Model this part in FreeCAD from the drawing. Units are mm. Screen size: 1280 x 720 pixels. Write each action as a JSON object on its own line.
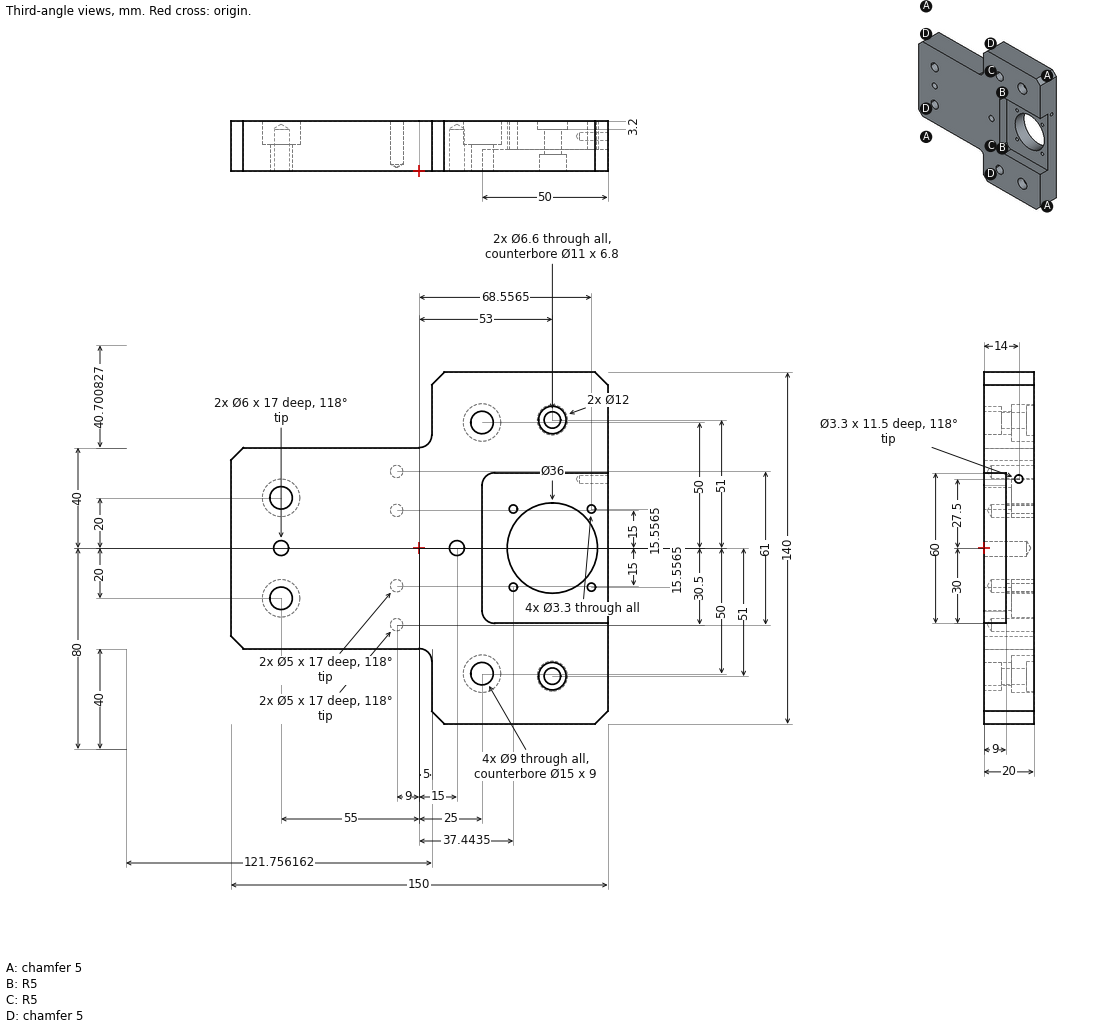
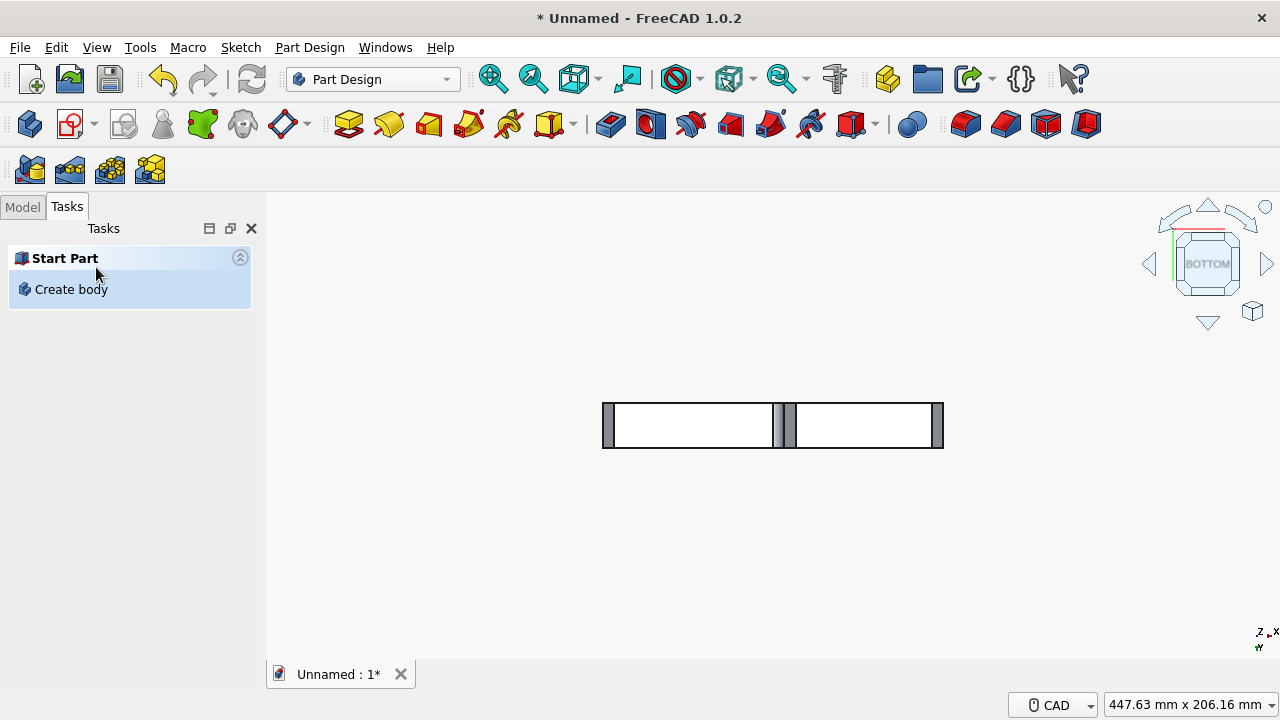
{"action": "left_click", "coordinate": [494, 80]}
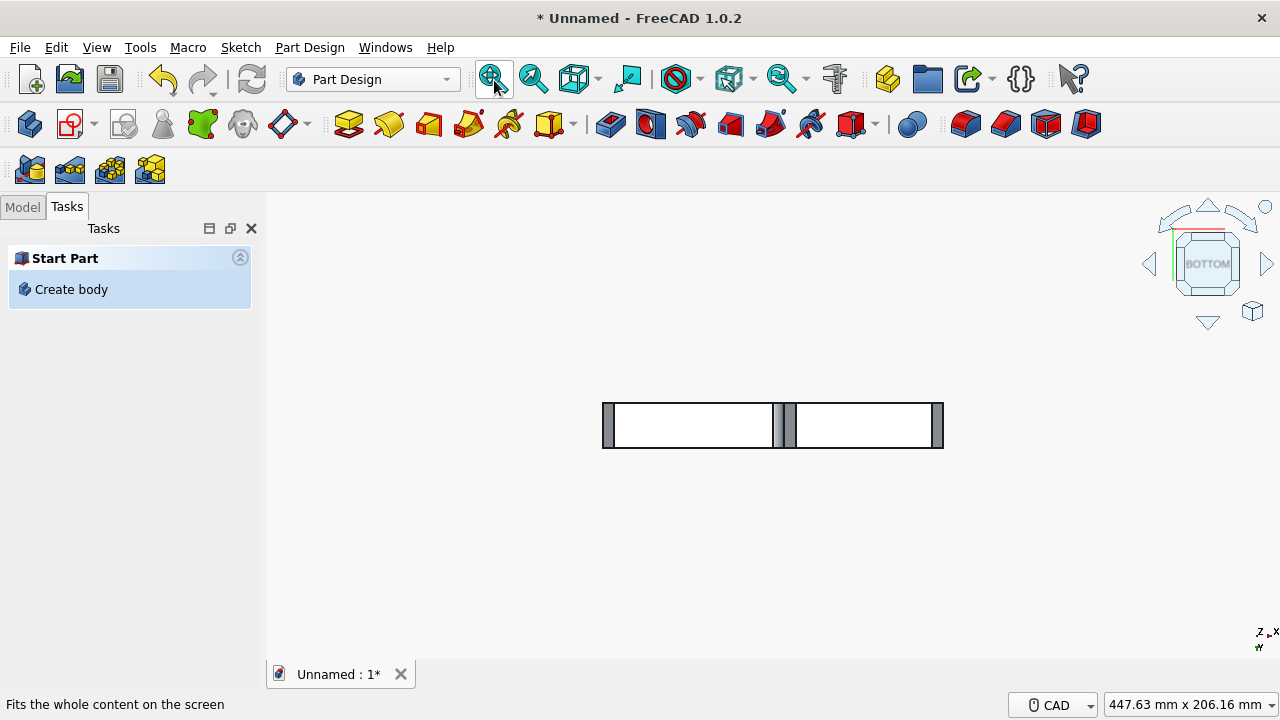
{"action": "key", "text": "4"}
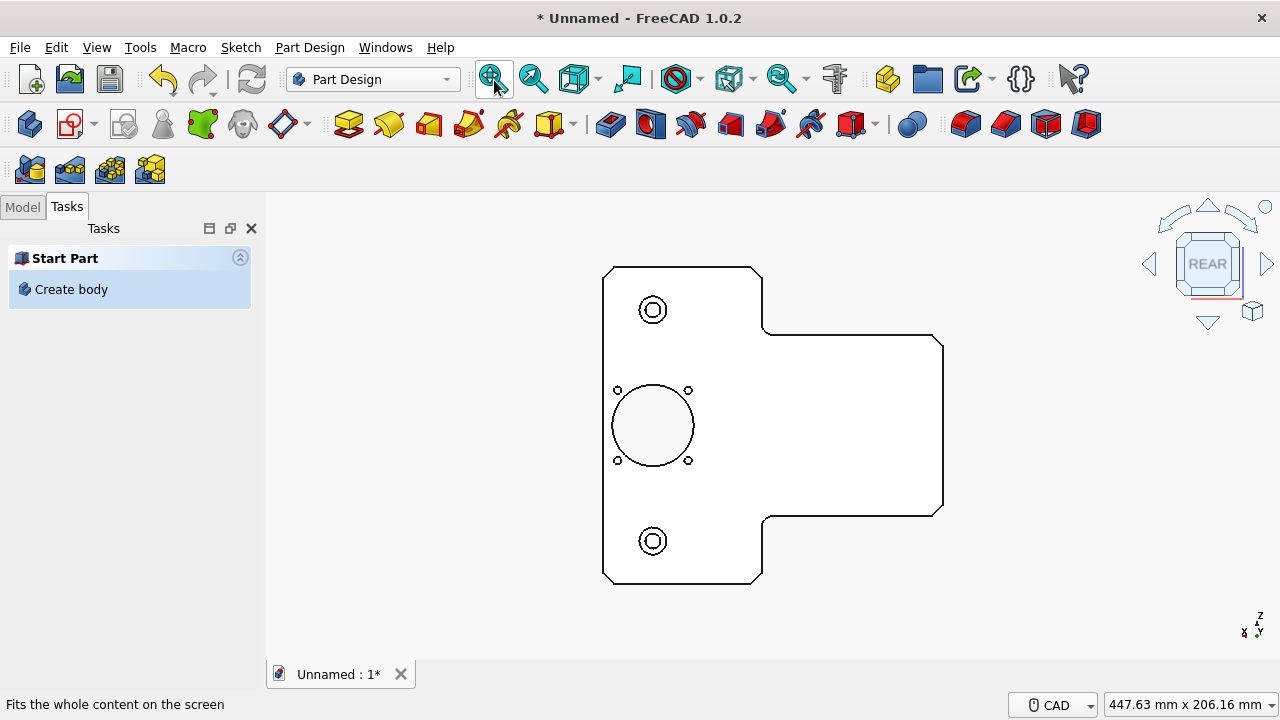
{"action": "left_click", "coordinate": [822, 424]}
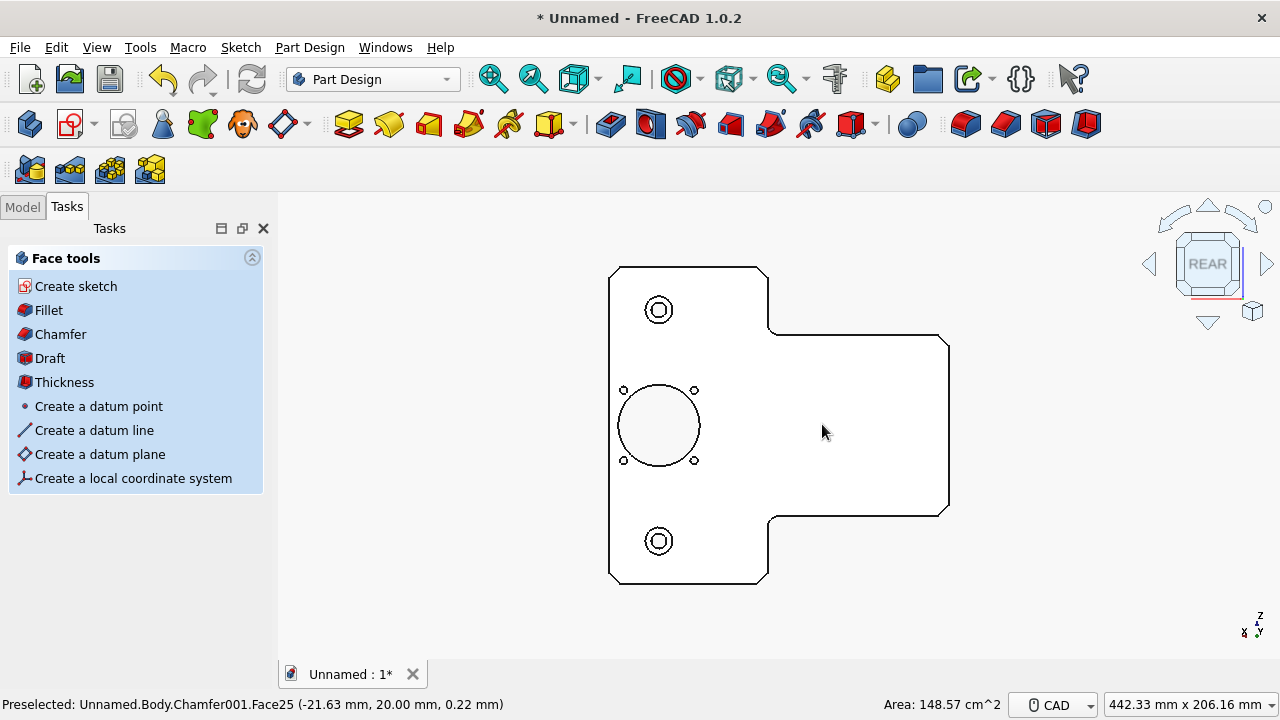
{"action": "left_click", "coordinate": [70, 124]}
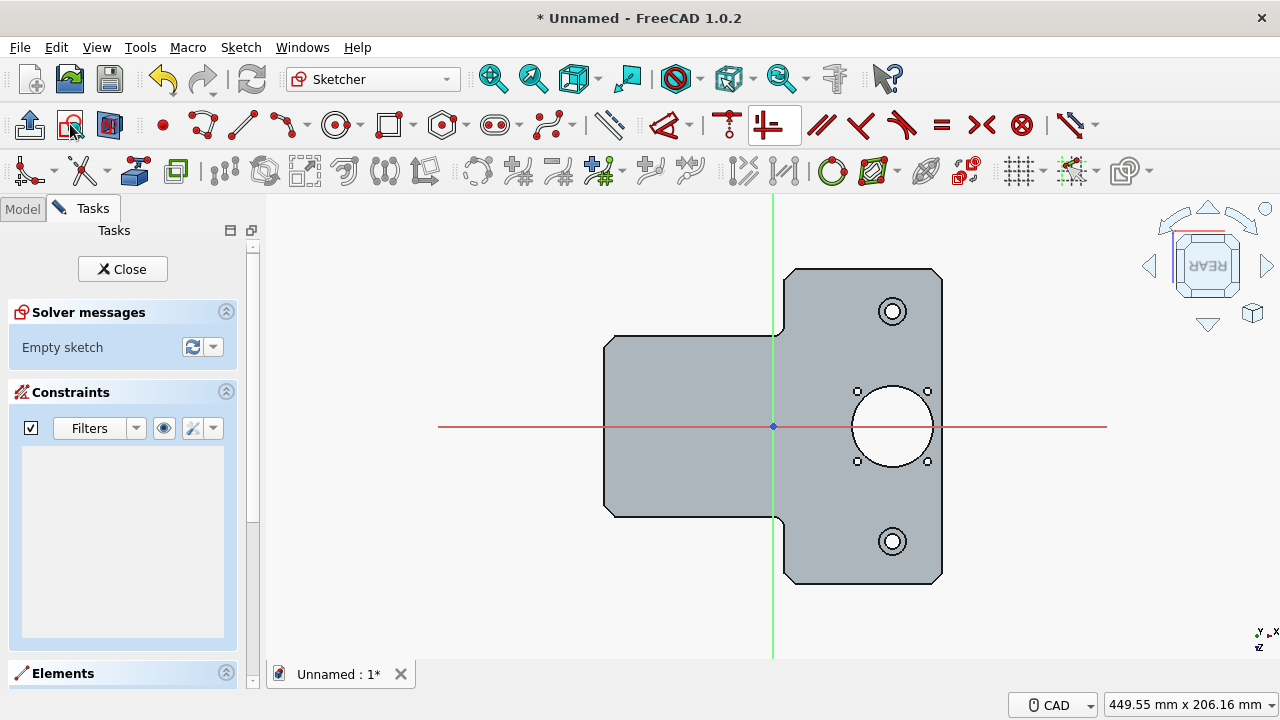
{"action": "left_click", "coordinate": [336, 126]}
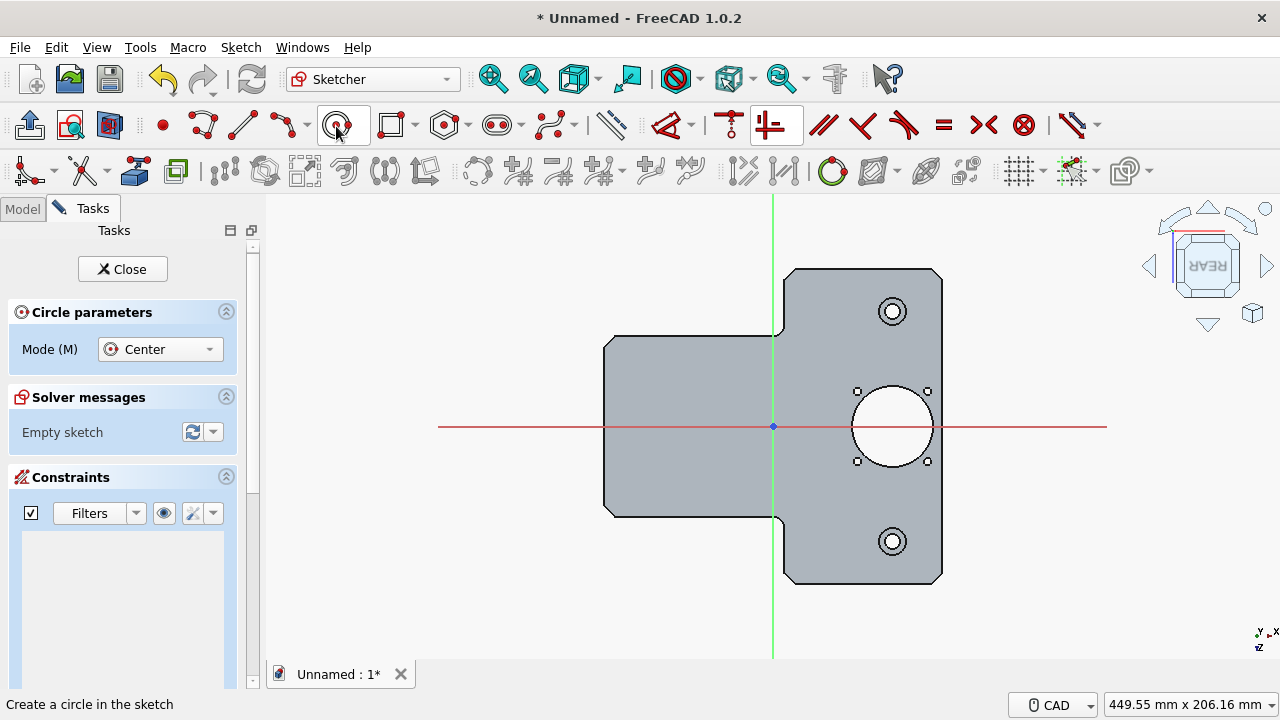
{"action": "scroll", "coordinate": [829, 314], "scroll_direction": "up", "scroll_amount": 5}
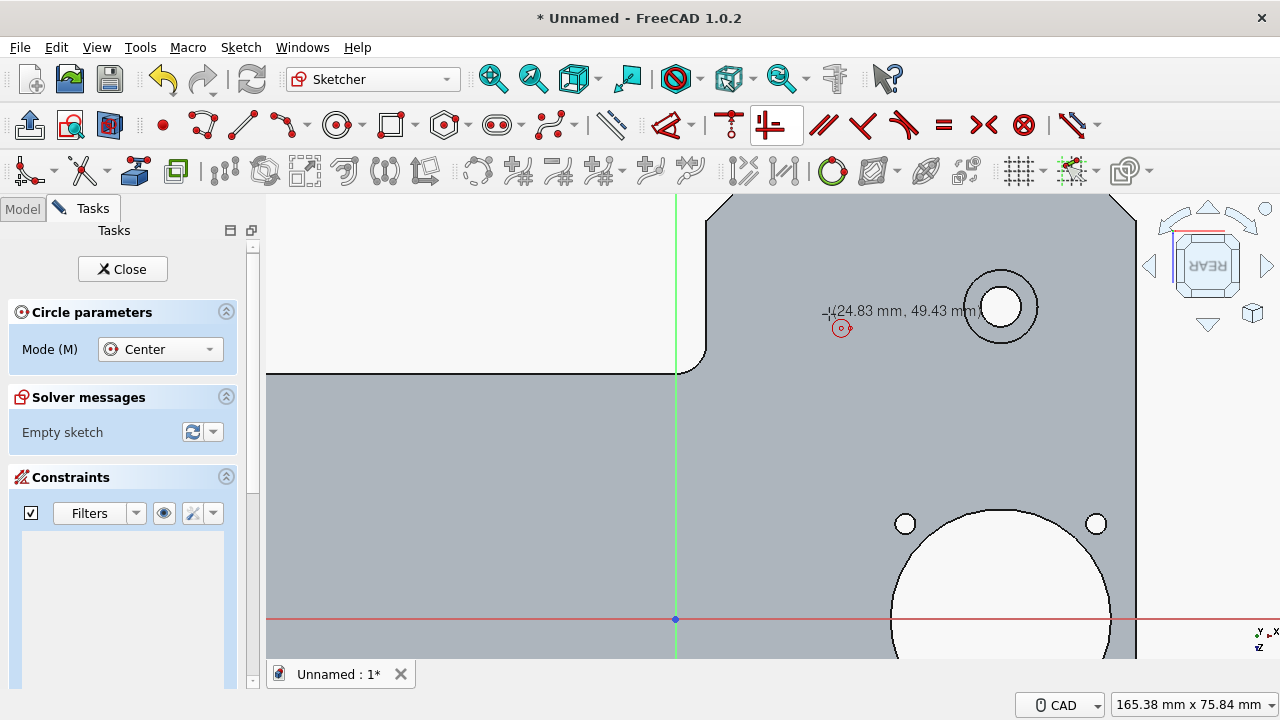
{"action": "left_click", "coordinate": [829, 313]}
{"action": "left_click", "coordinate": [849, 293]}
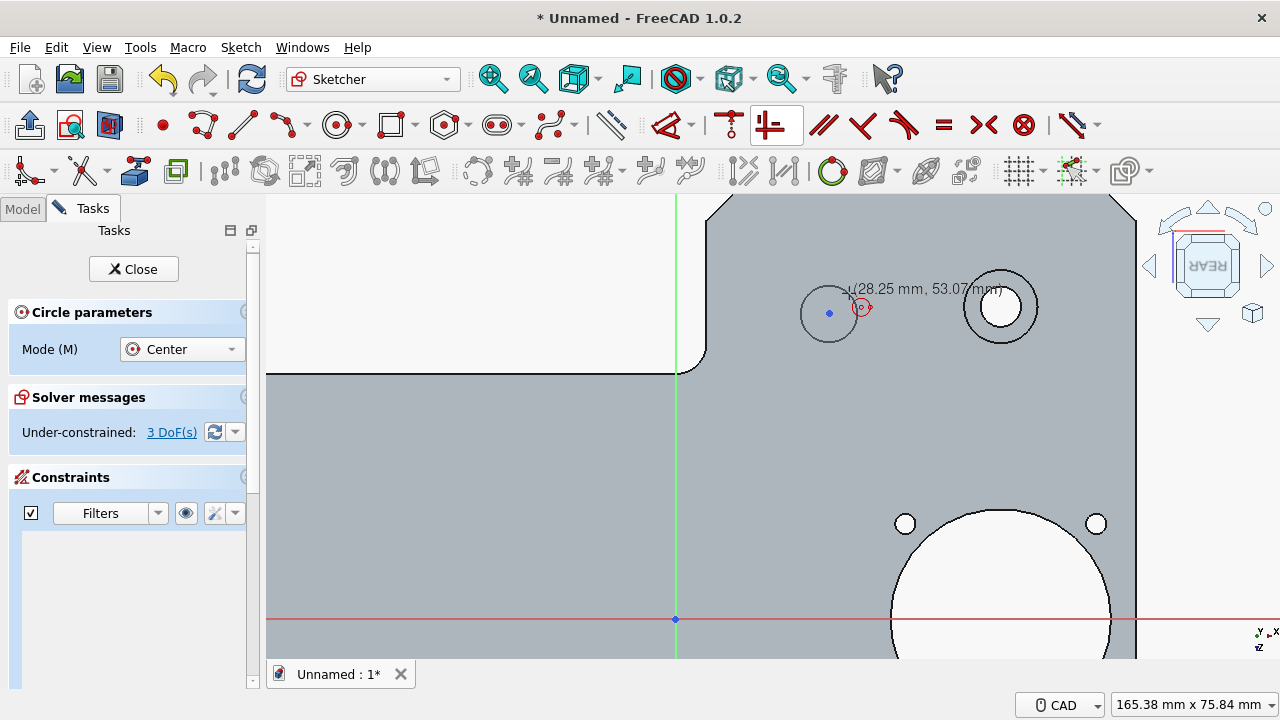
{"action": "scroll", "coordinate": [803, 269], "scroll_direction": "down", "scroll_amount": 4}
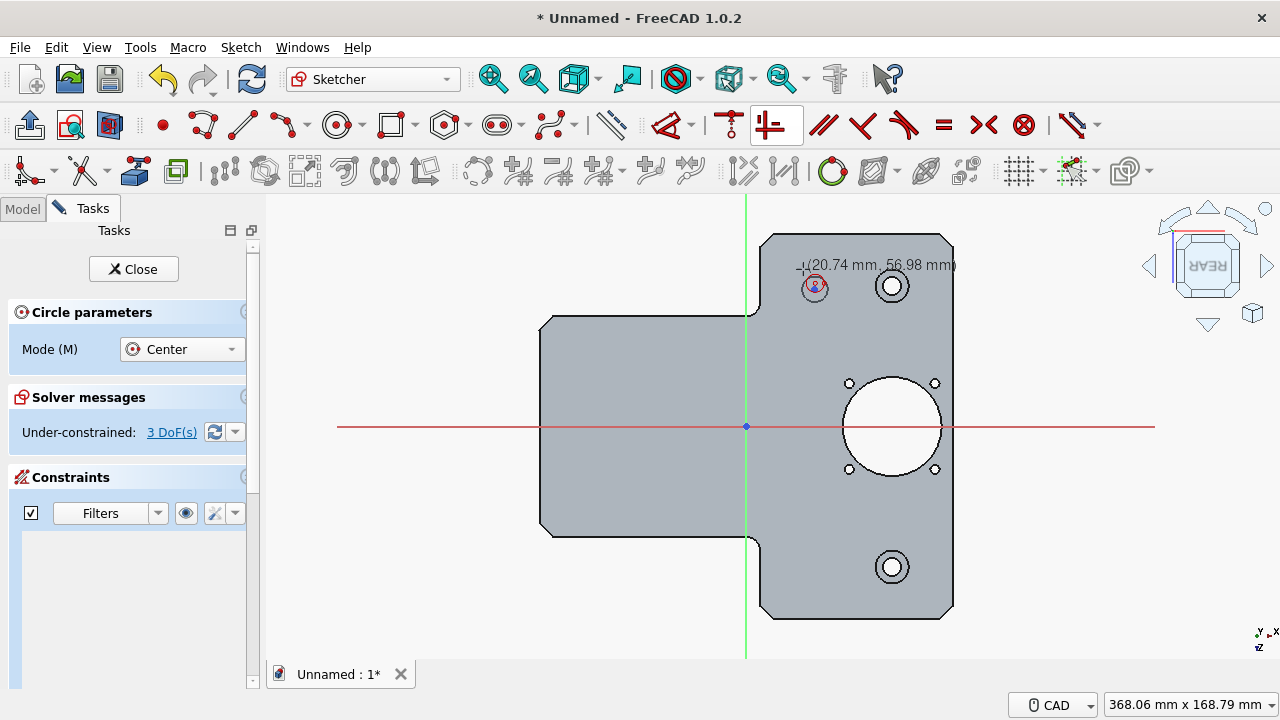
{"action": "scroll", "coordinate": [815, 564], "scroll_direction": "up", "scroll_amount": 4}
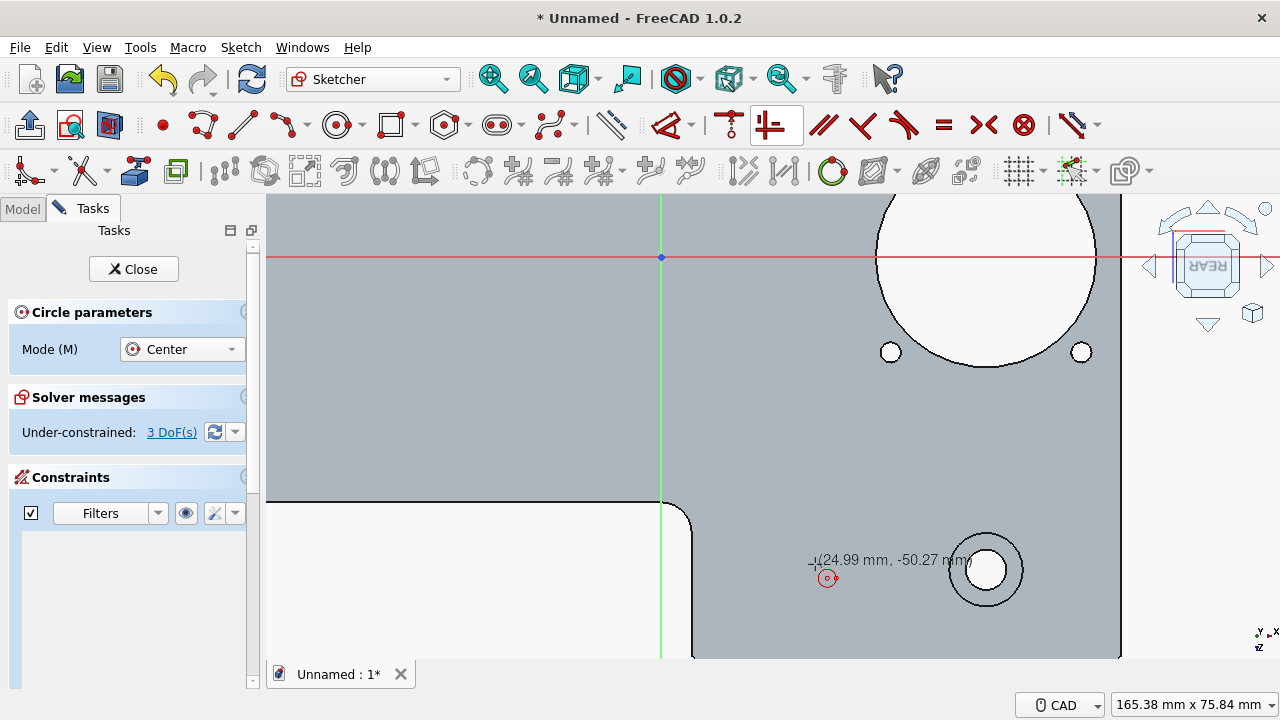
{"action": "left_click", "coordinate": [814, 564]}
{"action": "left_click", "coordinate": [834, 544]}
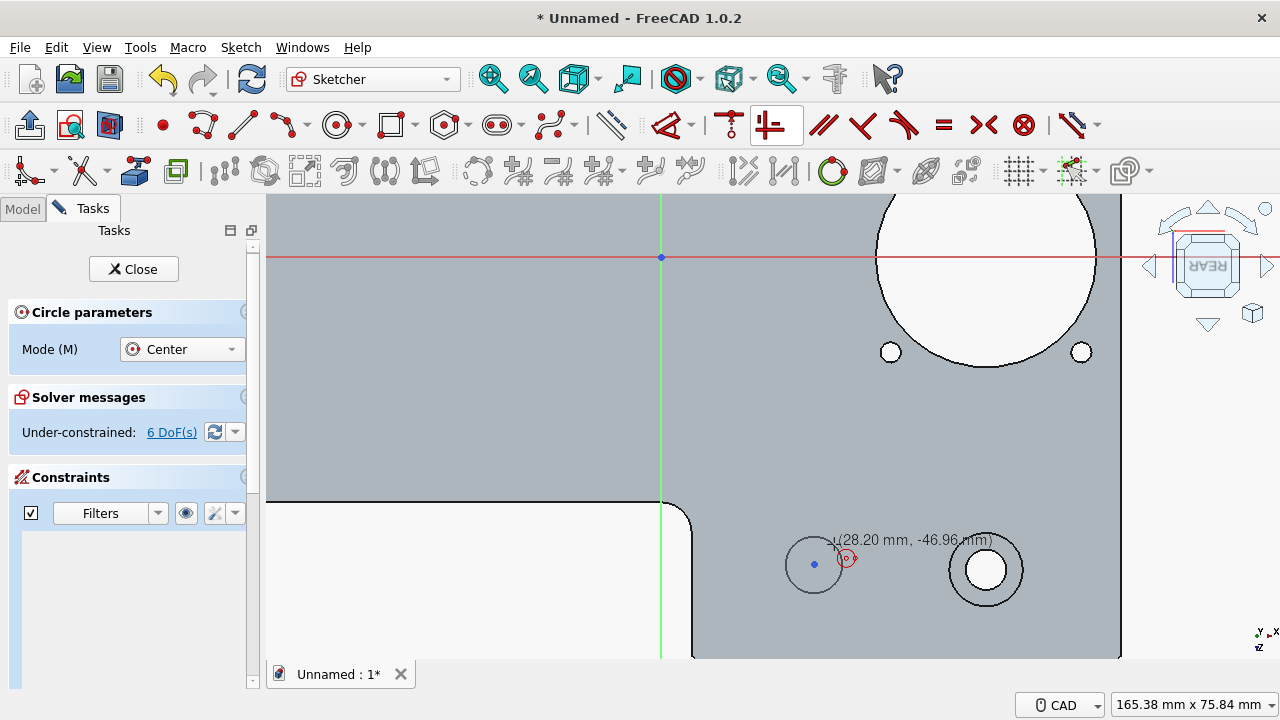
{"action": "scroll", "coordinate": [815, 565], "scroll_direction": "down", "scroll_amount": 4}